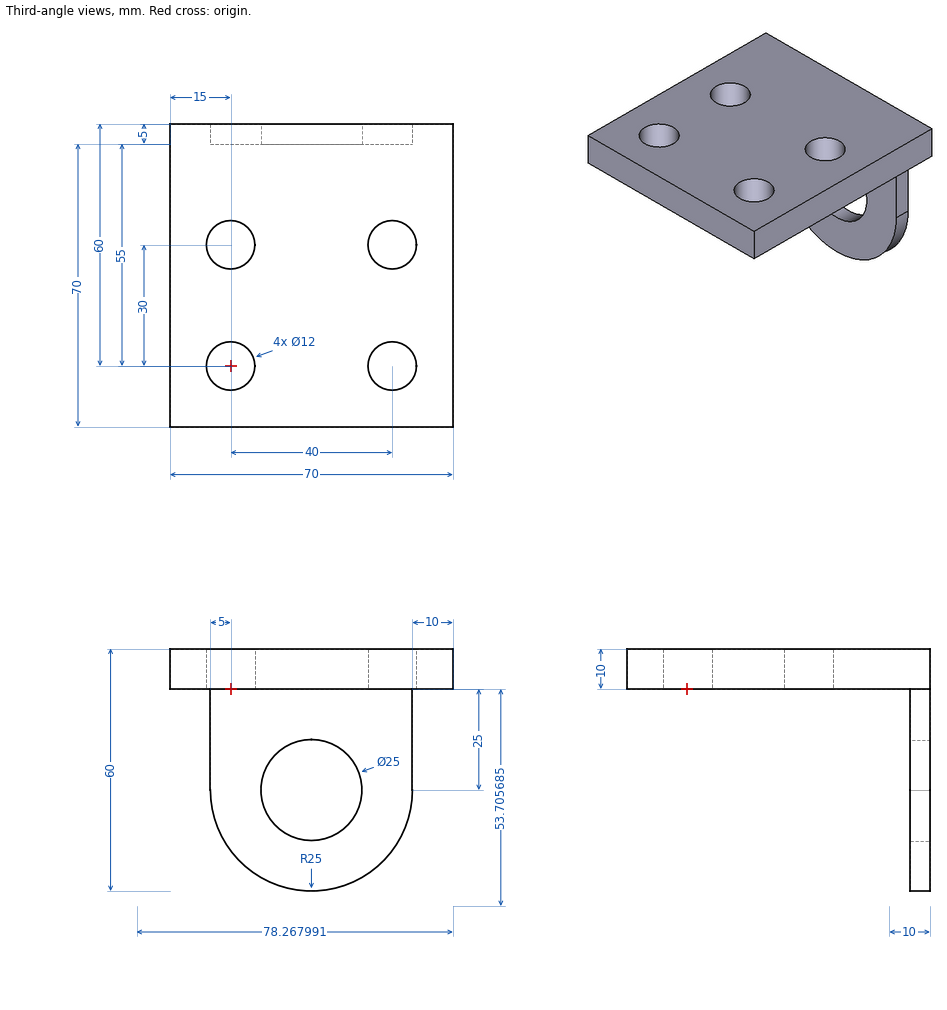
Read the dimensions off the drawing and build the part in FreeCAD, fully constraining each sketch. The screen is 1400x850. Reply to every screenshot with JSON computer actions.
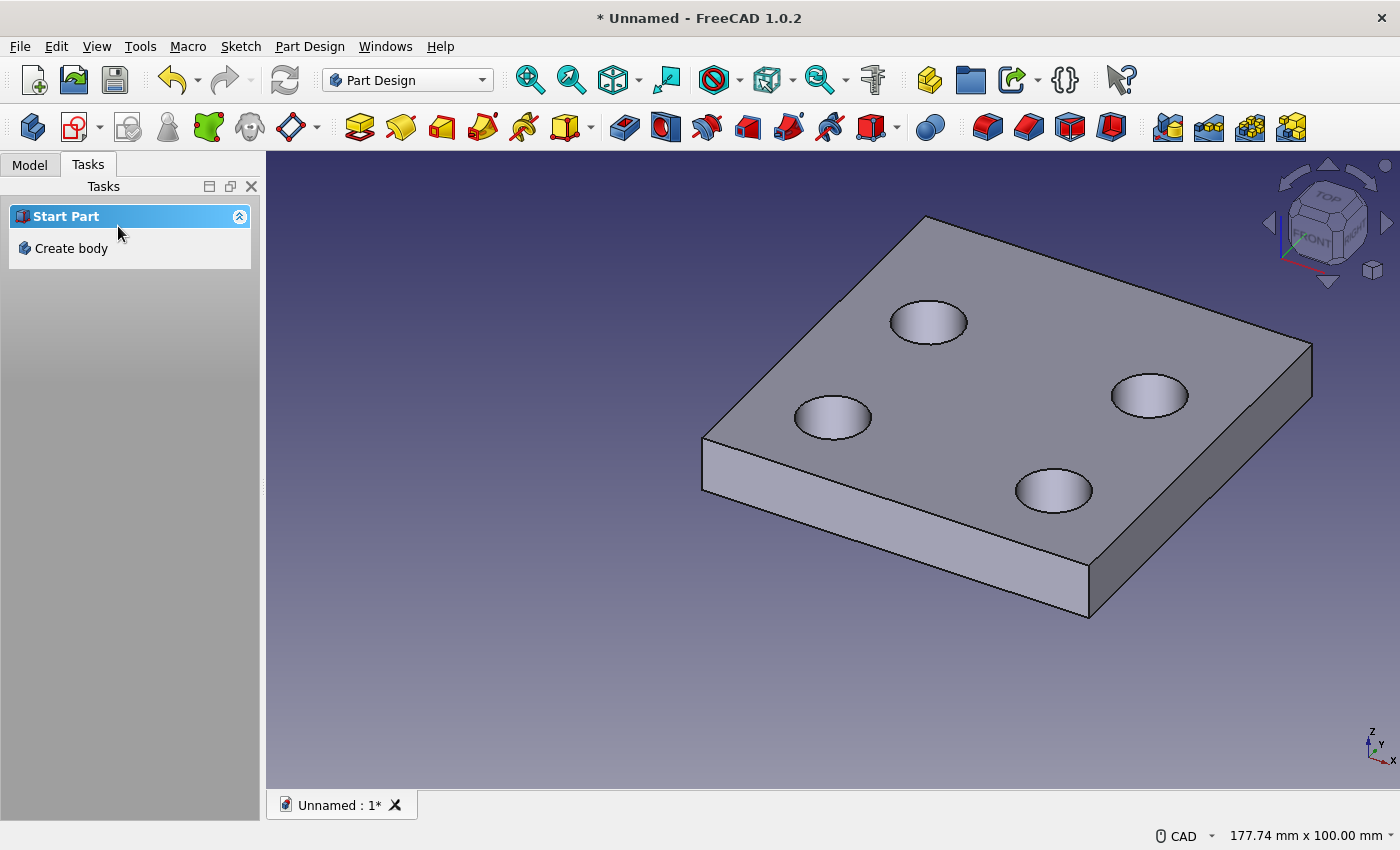
{"action": "left_click", "coordinate": [975, 422]}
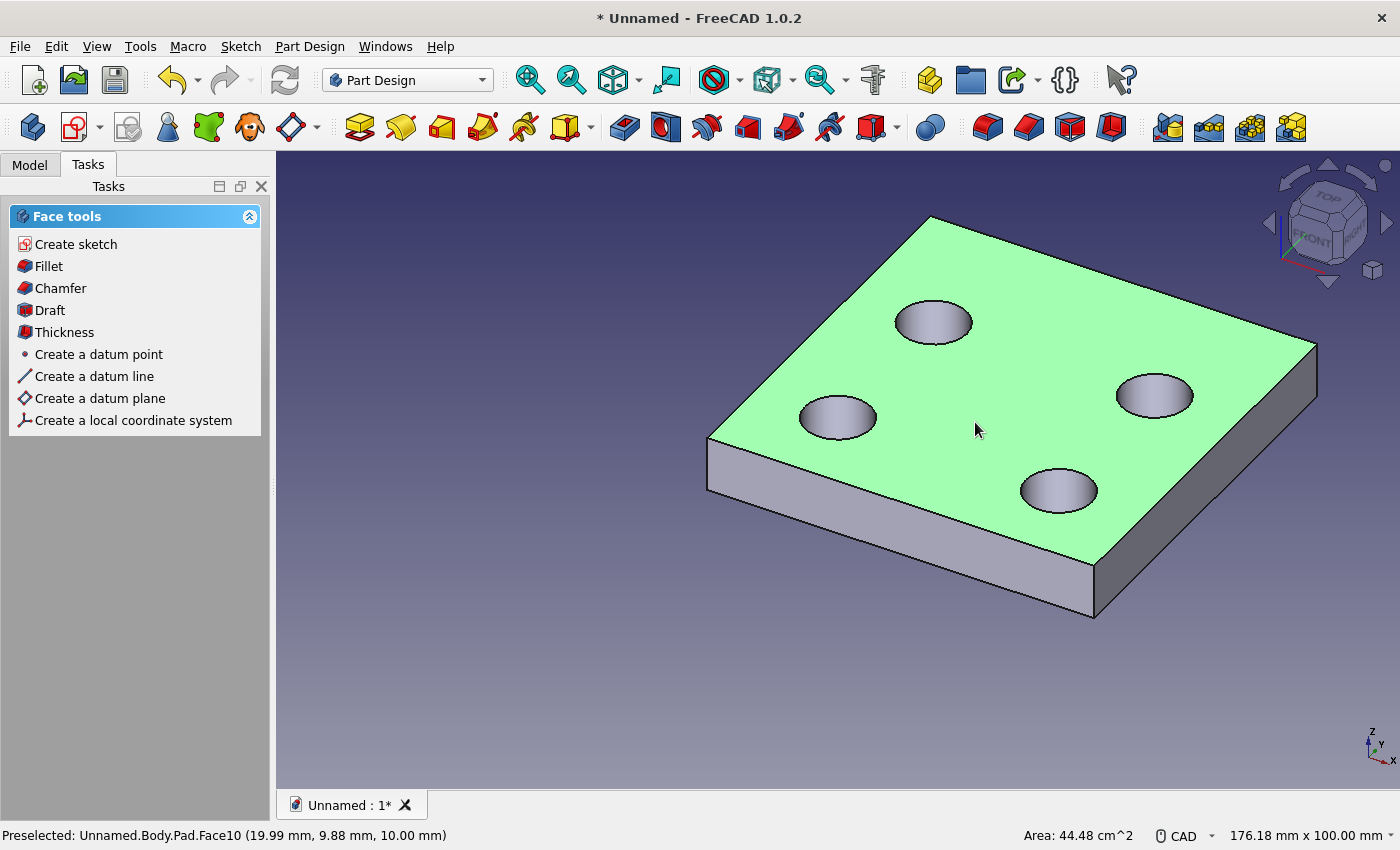
{"action": "left_click", "coordinate": [74, 128]}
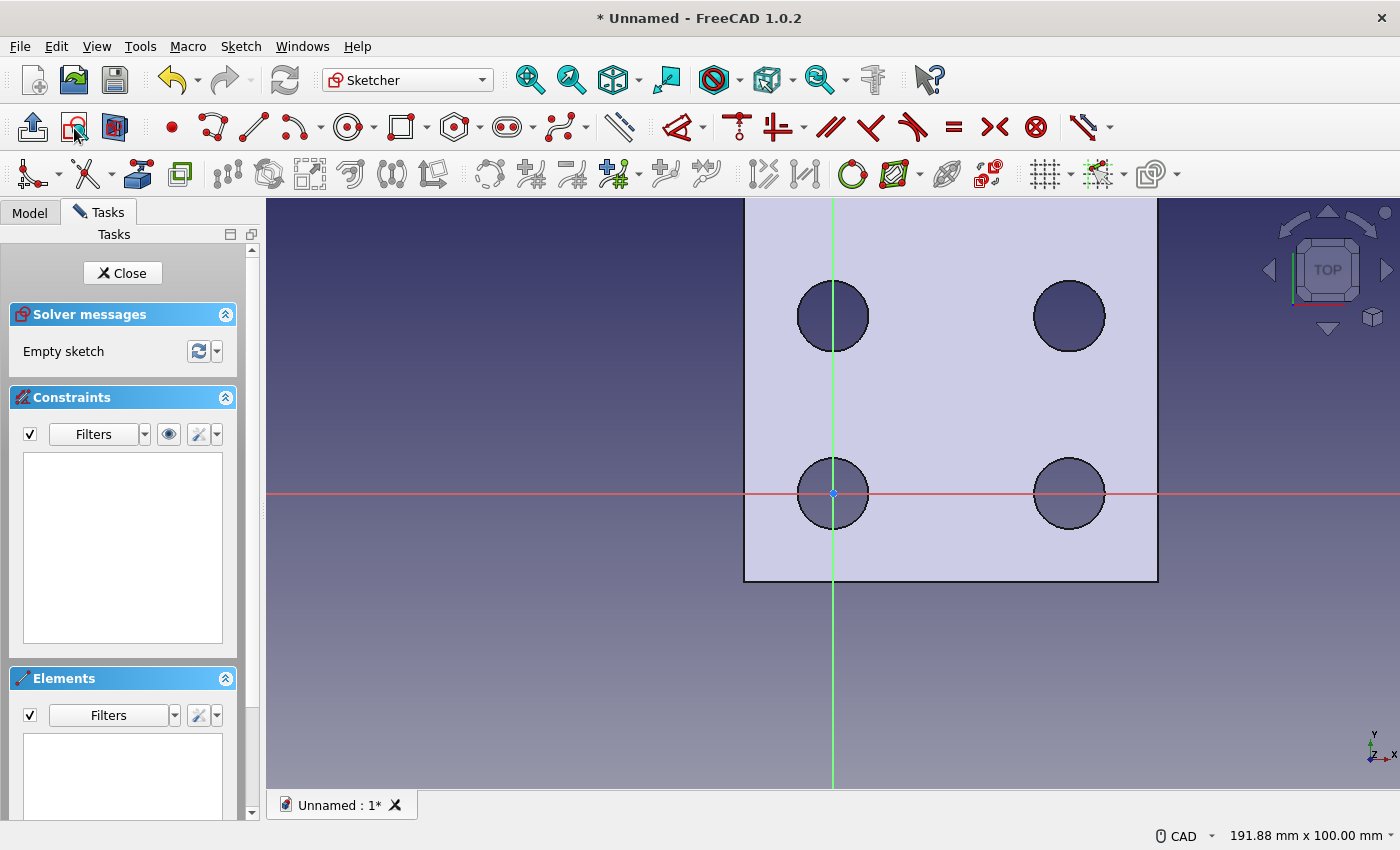
{"action": "scroll", "coordinate": [294, 761], "scroll_direction": "down", "scroll_amount": 1}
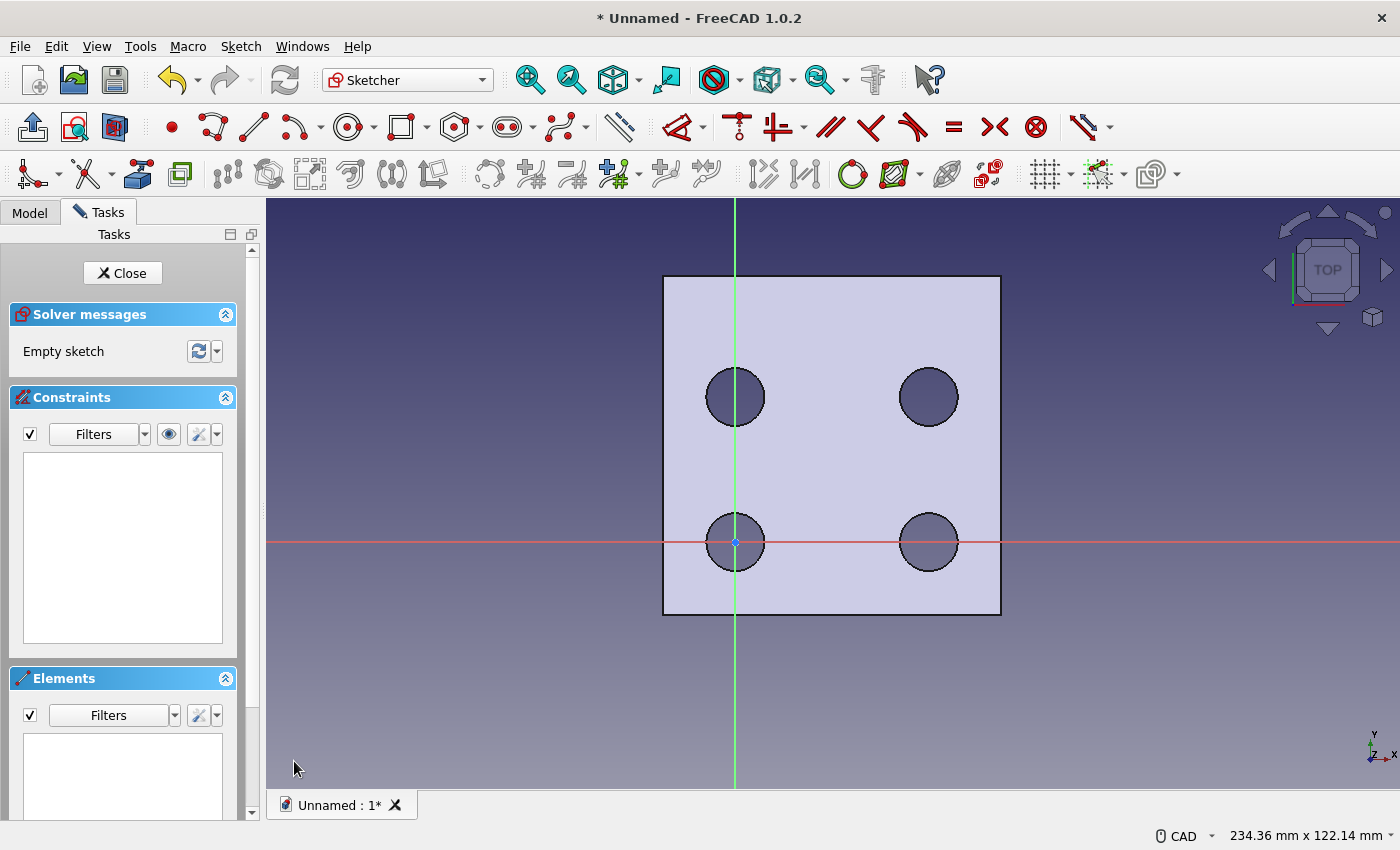
{"action": "left_click", "coordinate": [400, 128]}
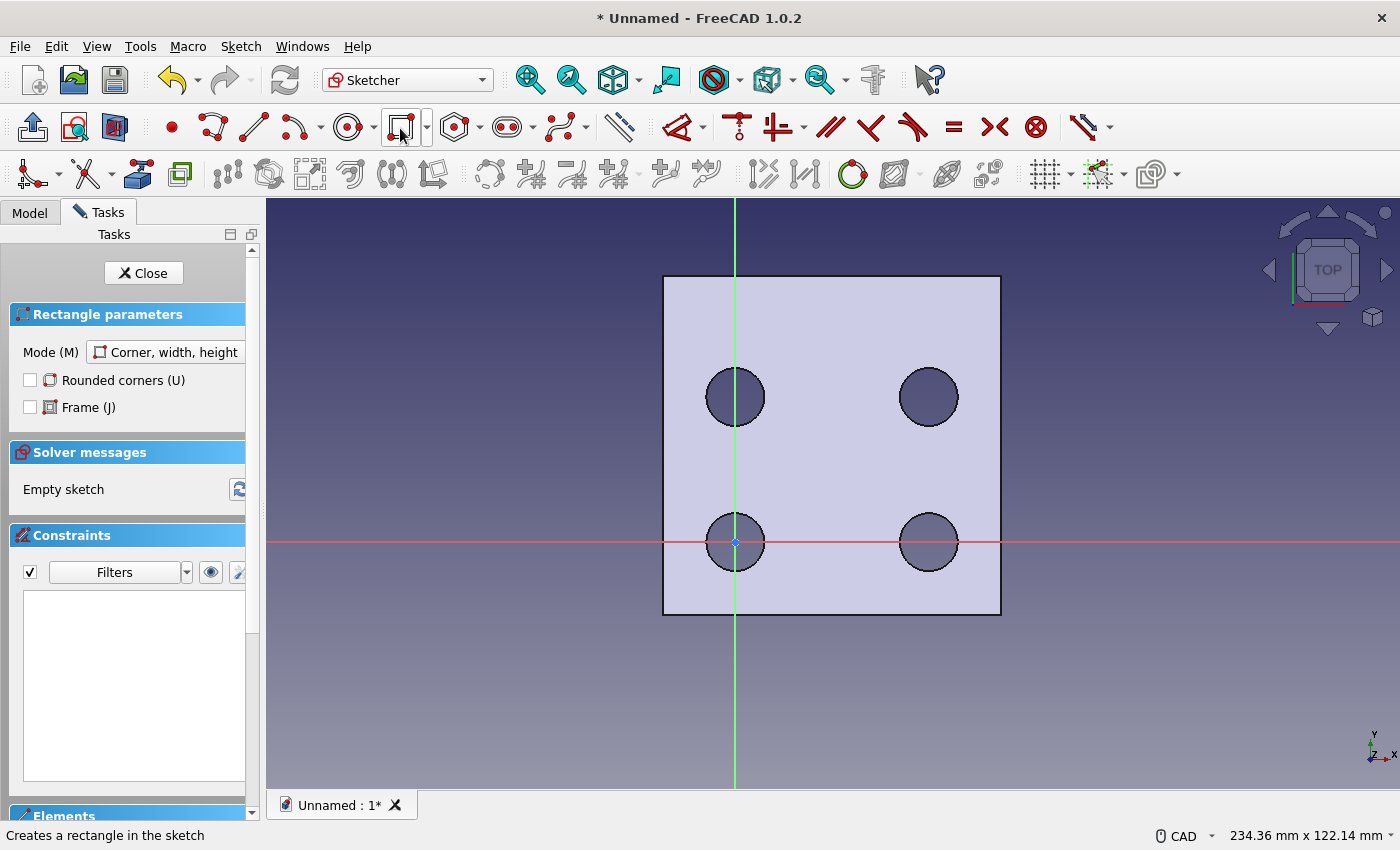
{"action": "left_click", "coordinate": [663, 252]}
{"action": "left_click", "coordinate": [1001, 276]}
{"action": "key", "text": "Escape"}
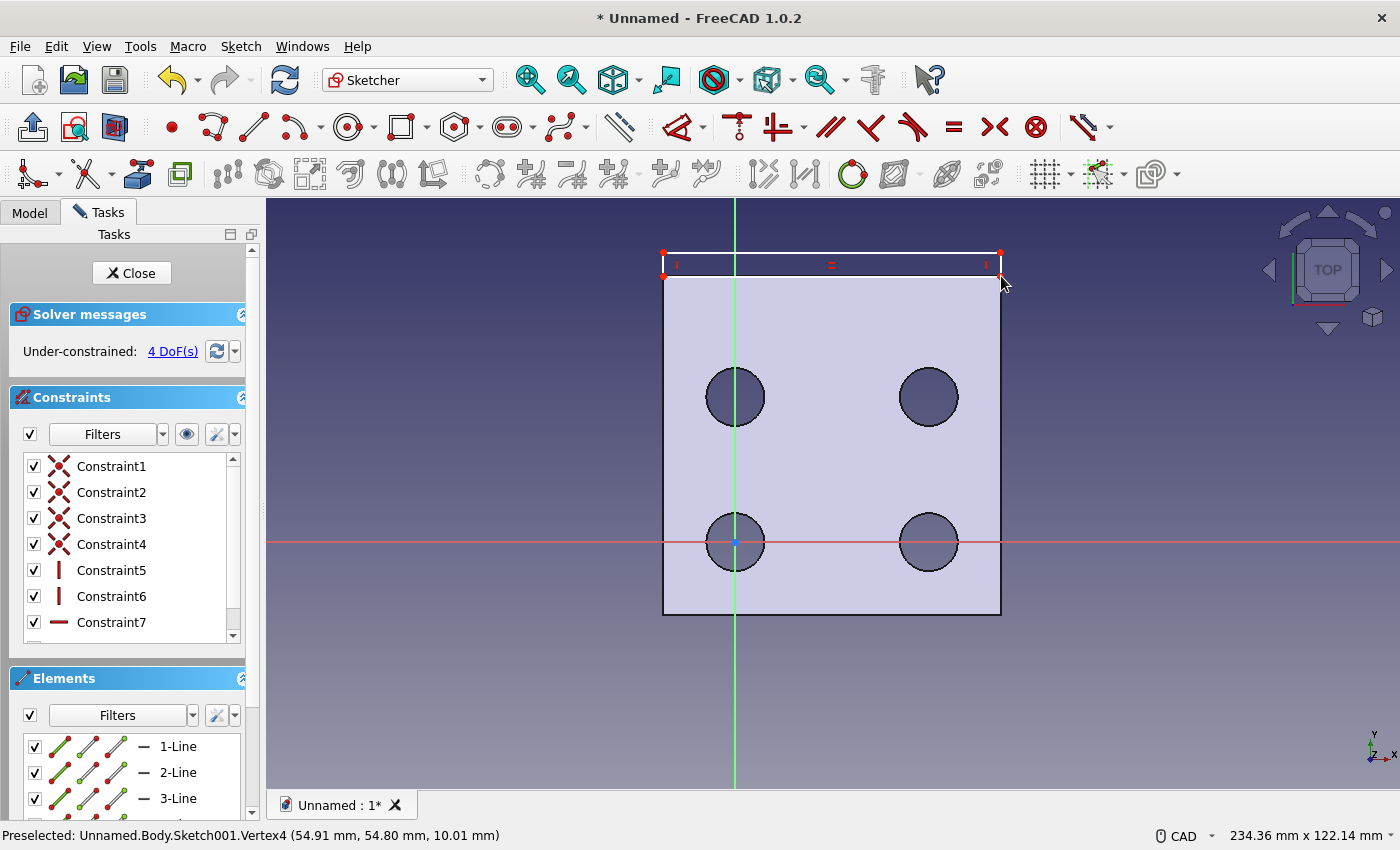
{"action": "left_click", "coordinate": [676, 128]}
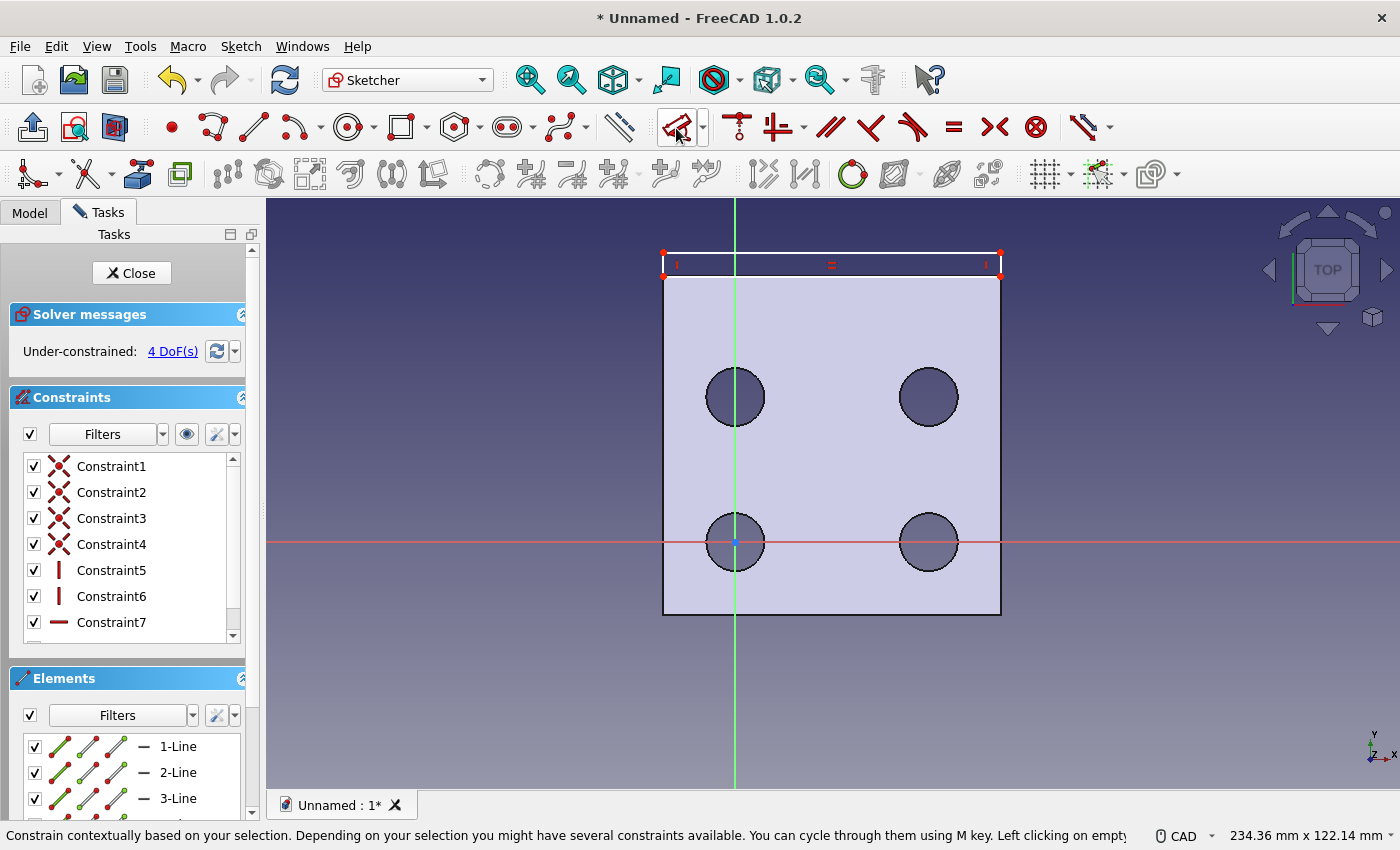
{"action": "scroll", "coordinate": [663, 263], "scroll_direction": "up", "scroll_amount": 3}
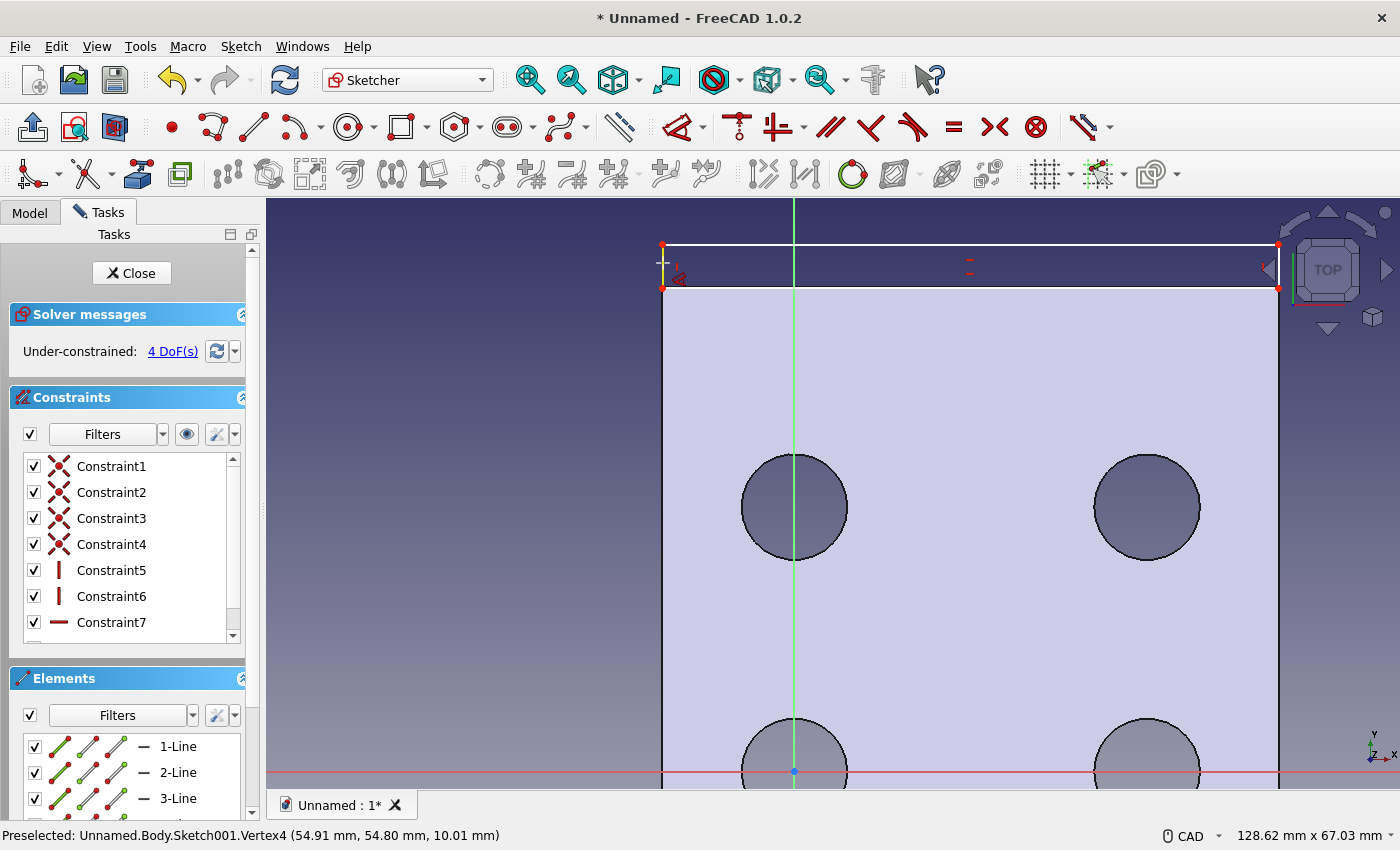
{"action": "left_click", "coordinate": [663, 262]}
{"action": "left_click", "coordinate": [629, 267]}